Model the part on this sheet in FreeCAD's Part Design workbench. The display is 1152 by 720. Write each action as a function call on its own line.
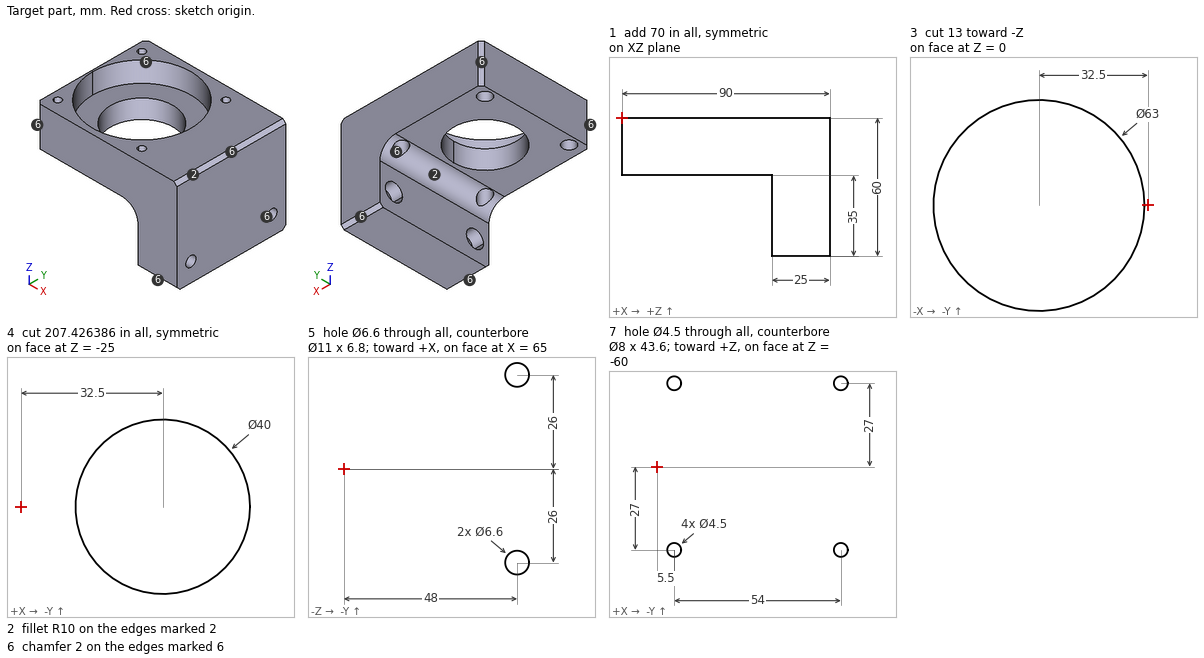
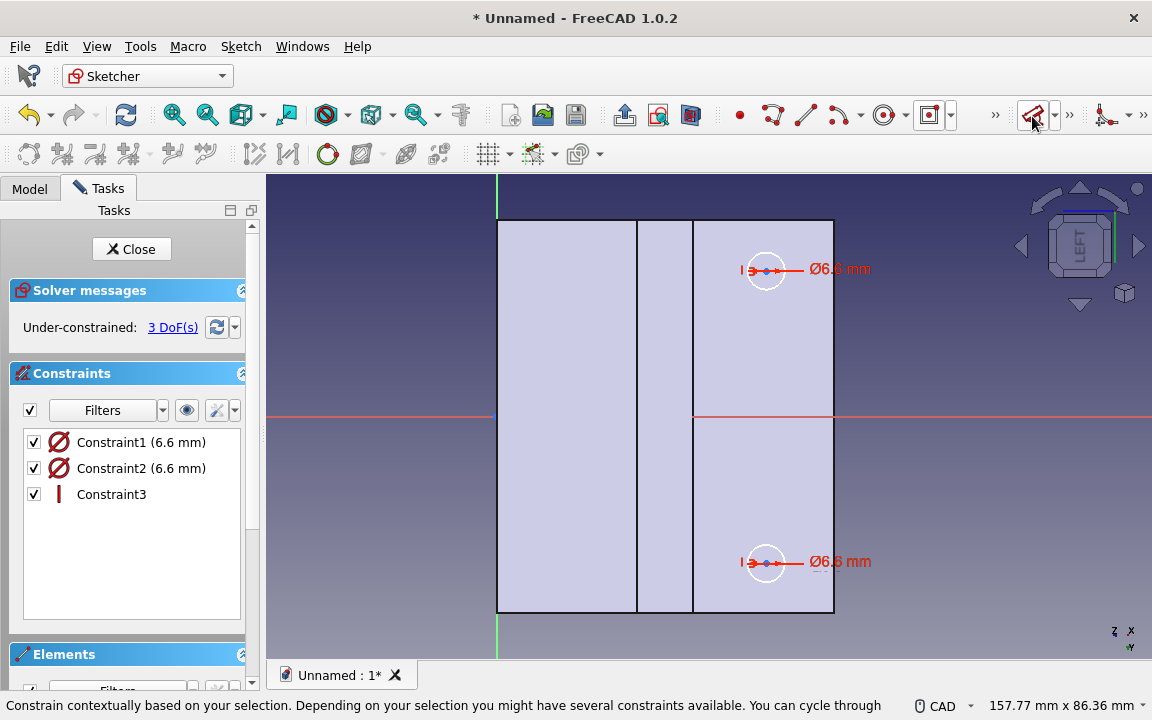
click(766, 564)
click(631, 598)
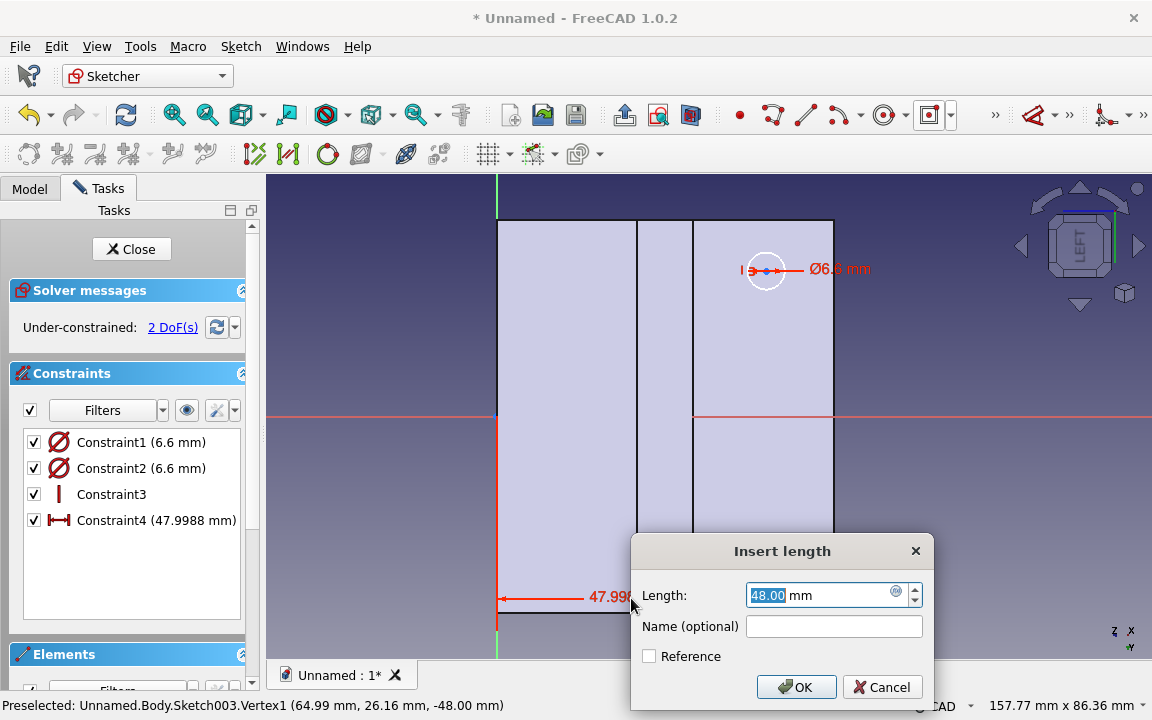
text(48)
key(Return)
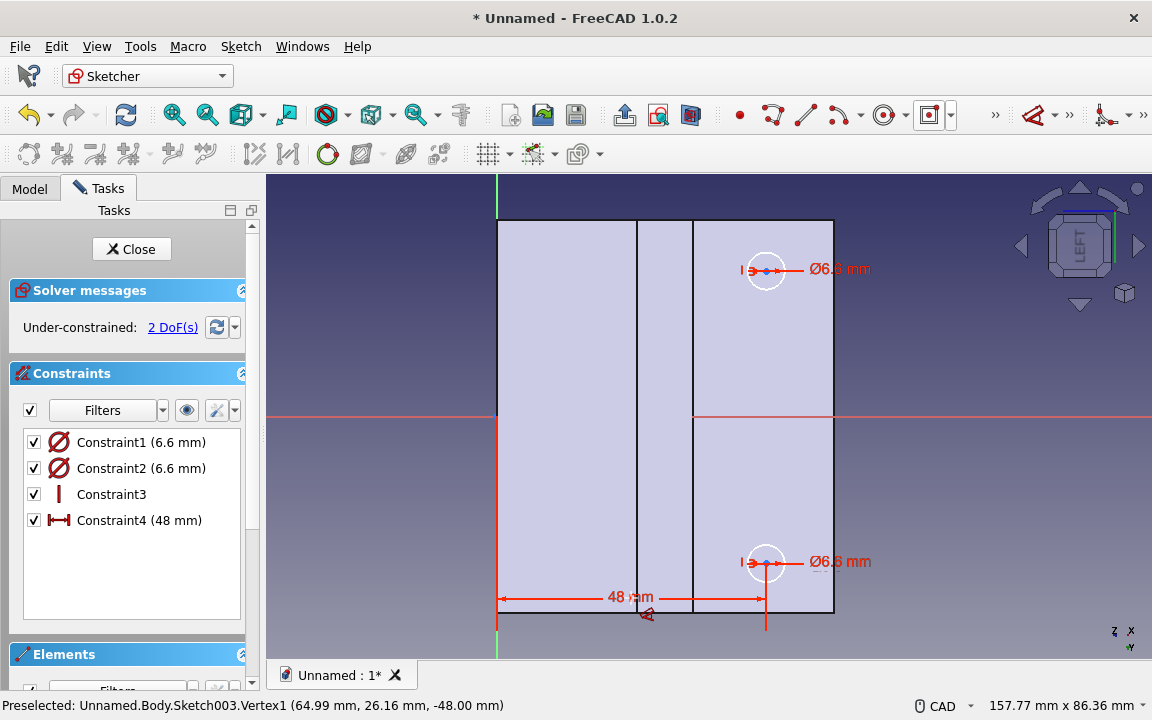
click(766, 564)
click(463, 490)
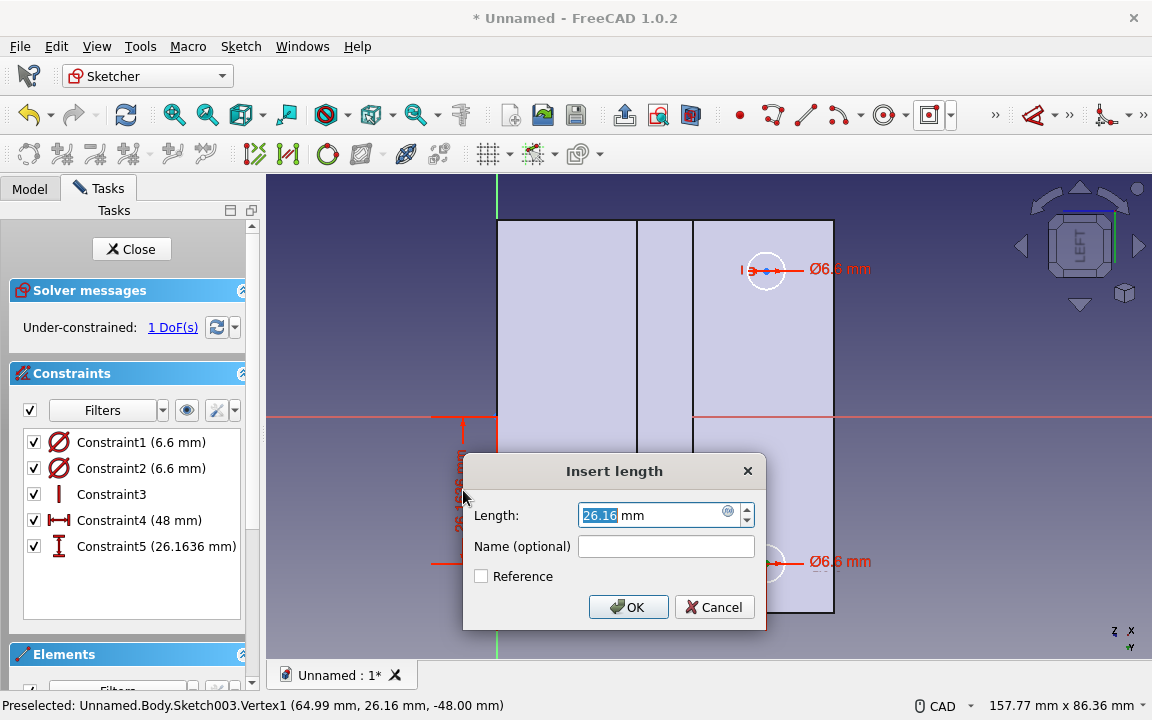
text(26)
key(Return)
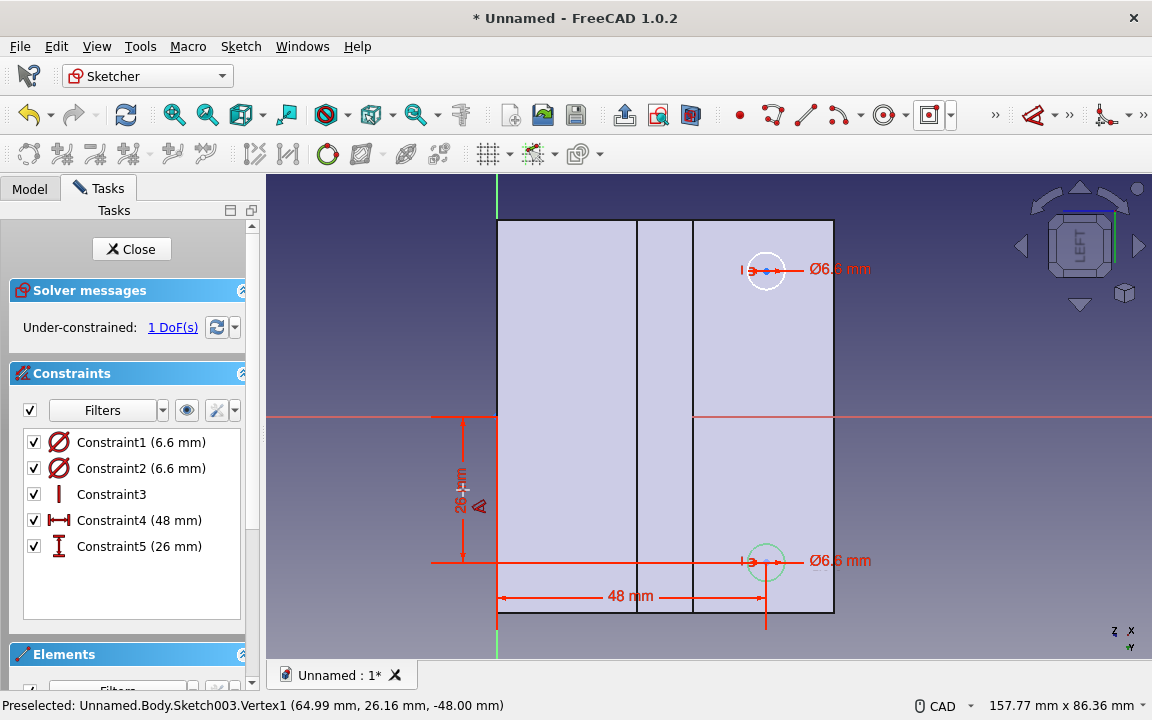
click(766, 271)
click(463, 344)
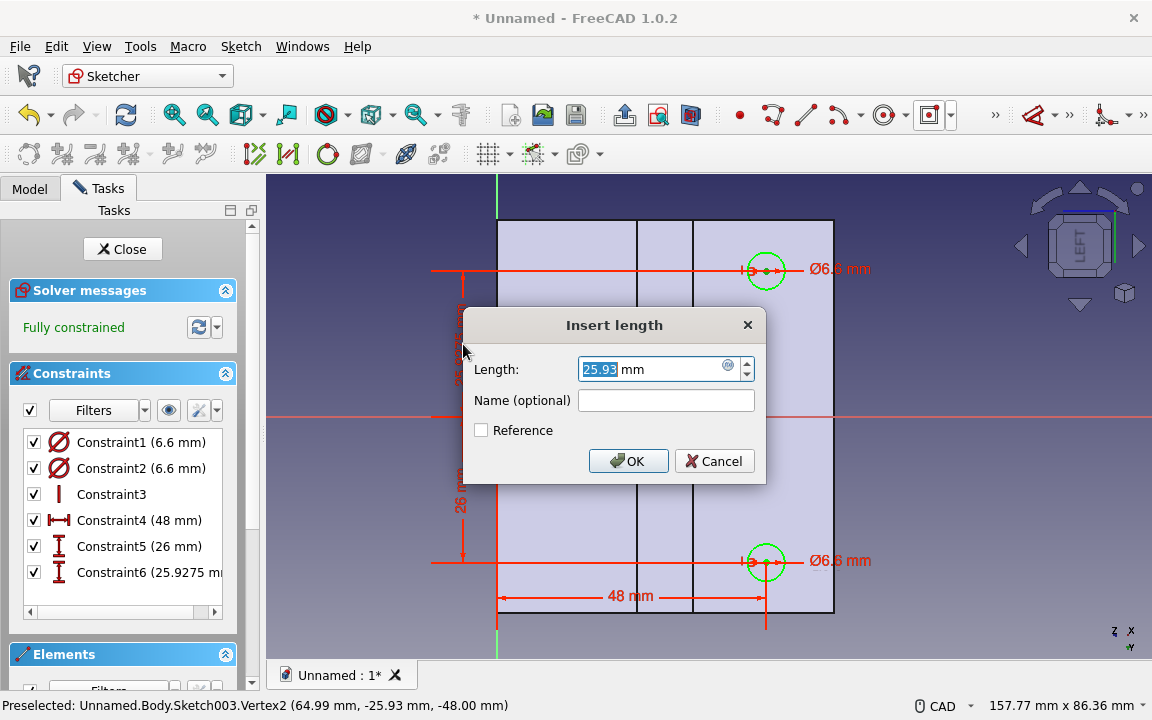
text(26)
key(Return)
key(Escape)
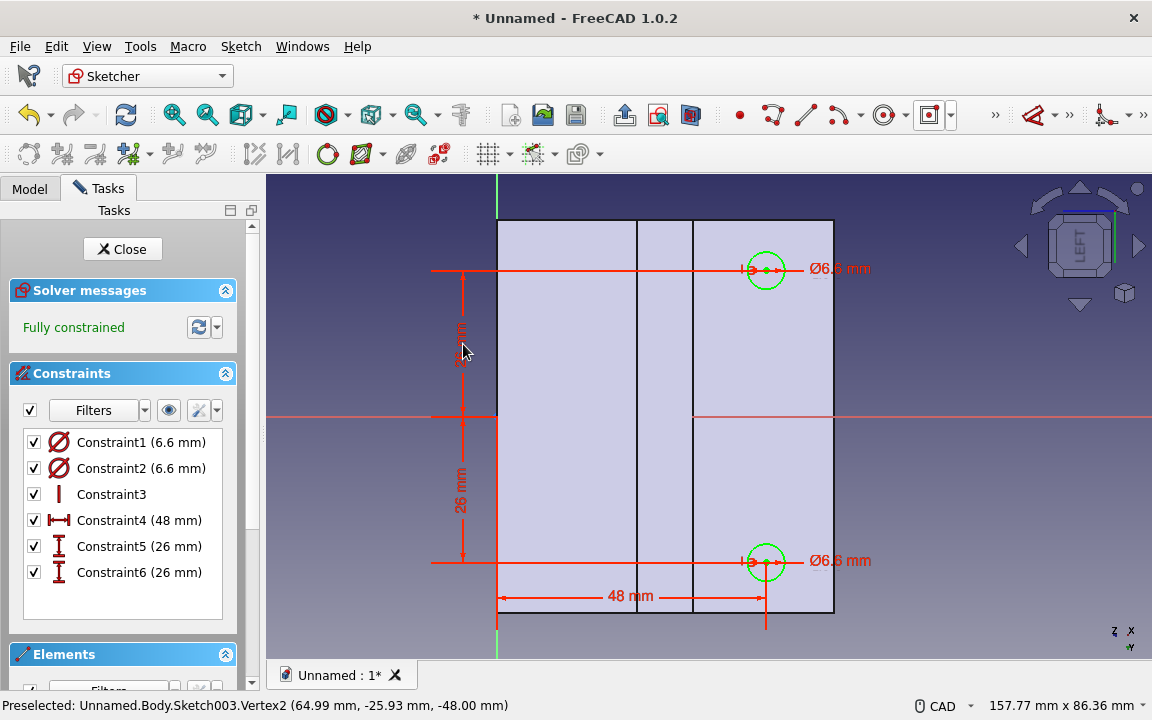
click(123, 249)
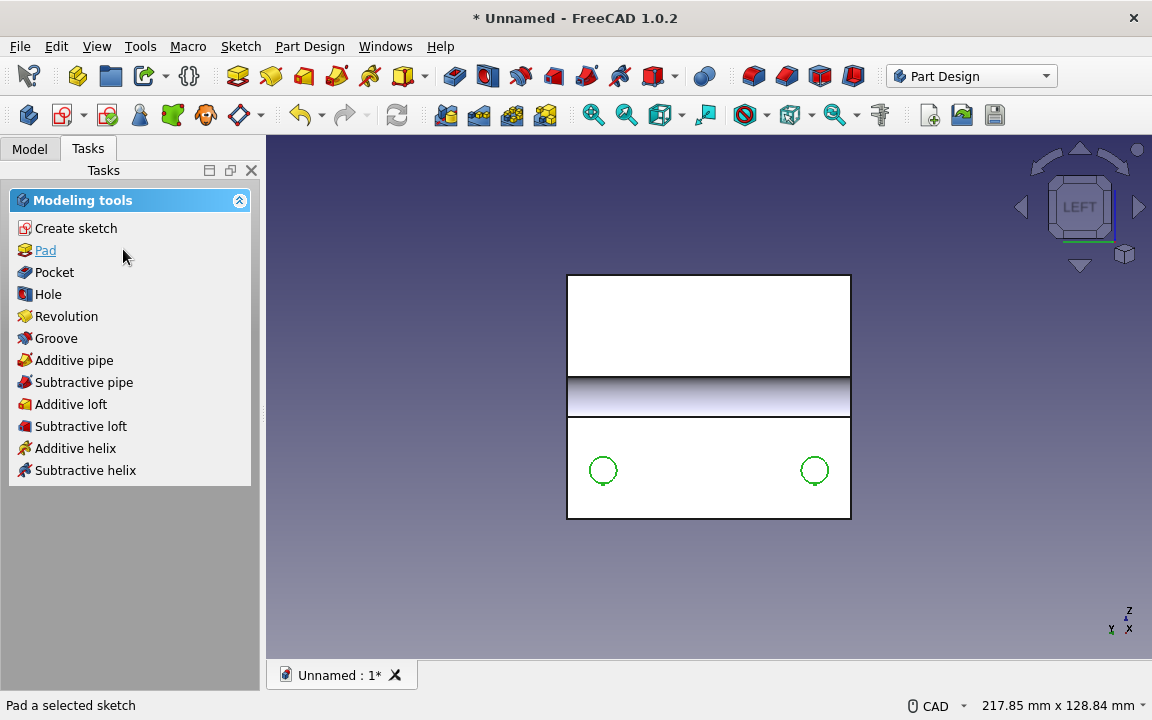
click(488, 76)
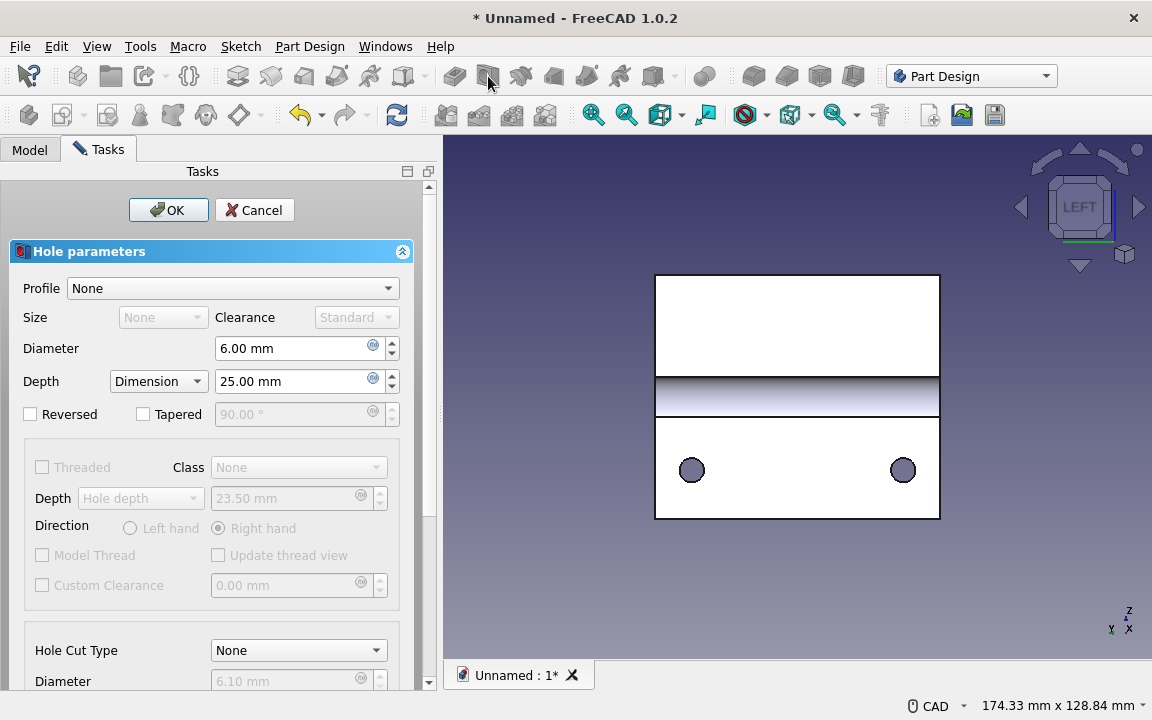
triple_click(300, 348)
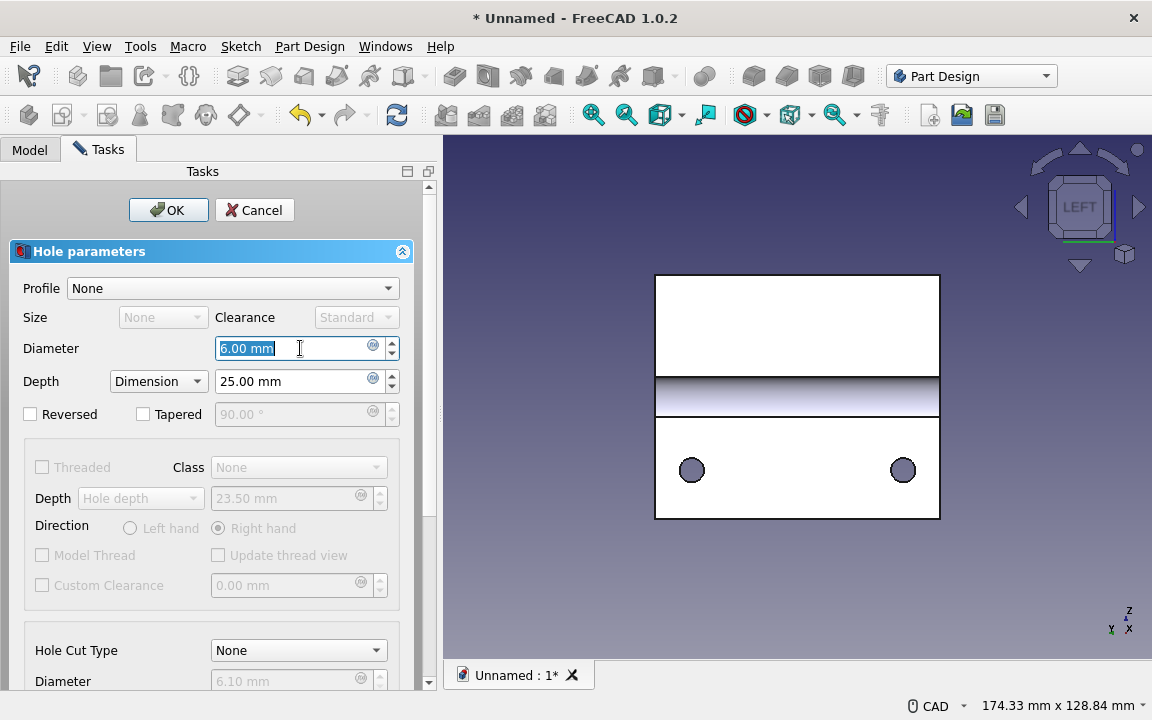
text(6.6)
key(Tab)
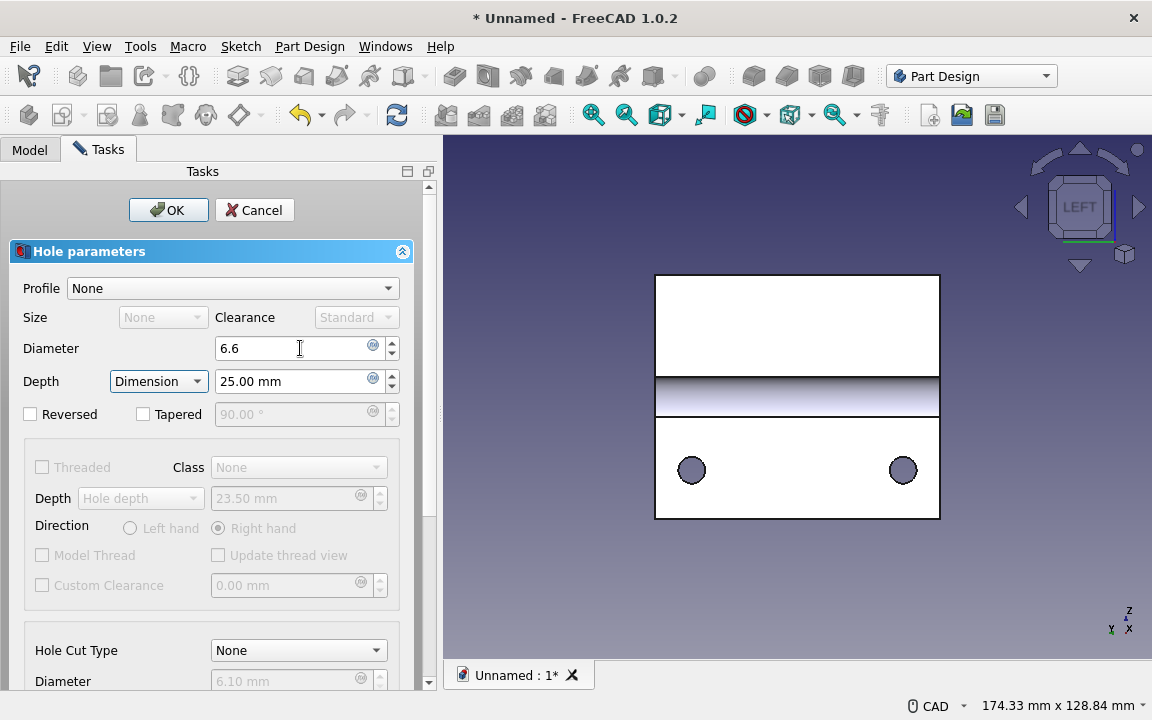
click(160, 382)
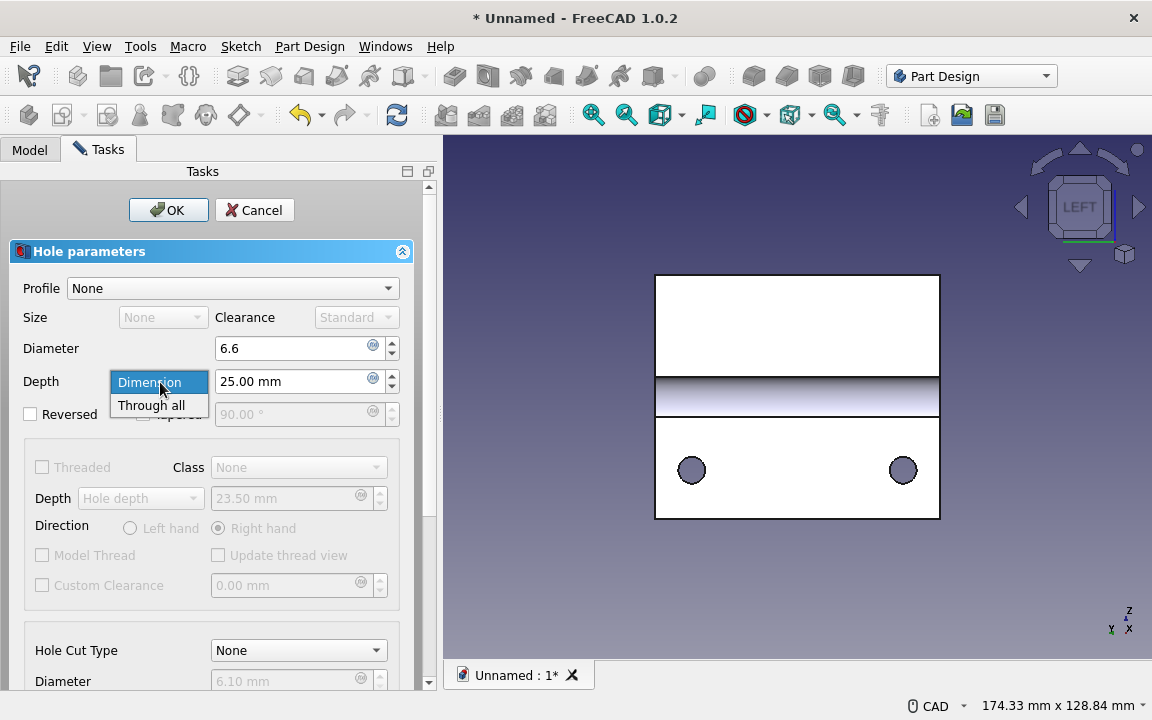
click(158, 406)